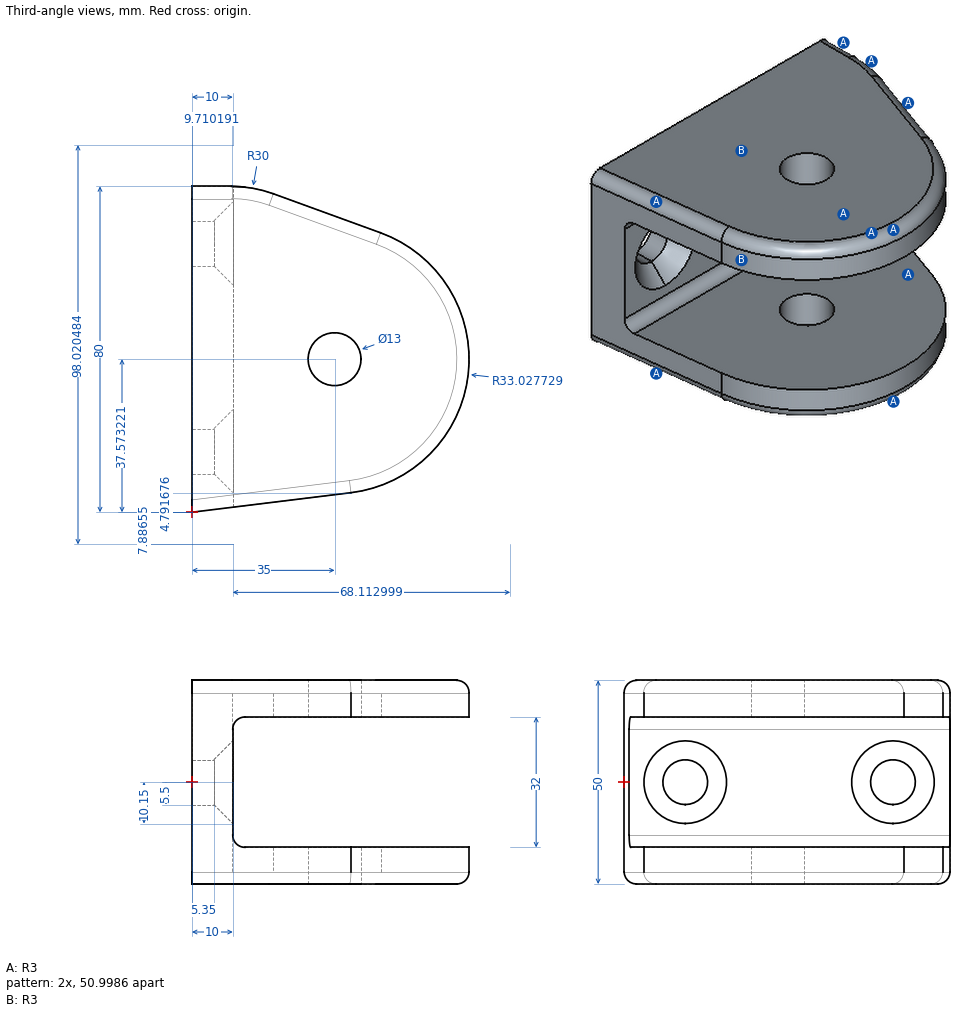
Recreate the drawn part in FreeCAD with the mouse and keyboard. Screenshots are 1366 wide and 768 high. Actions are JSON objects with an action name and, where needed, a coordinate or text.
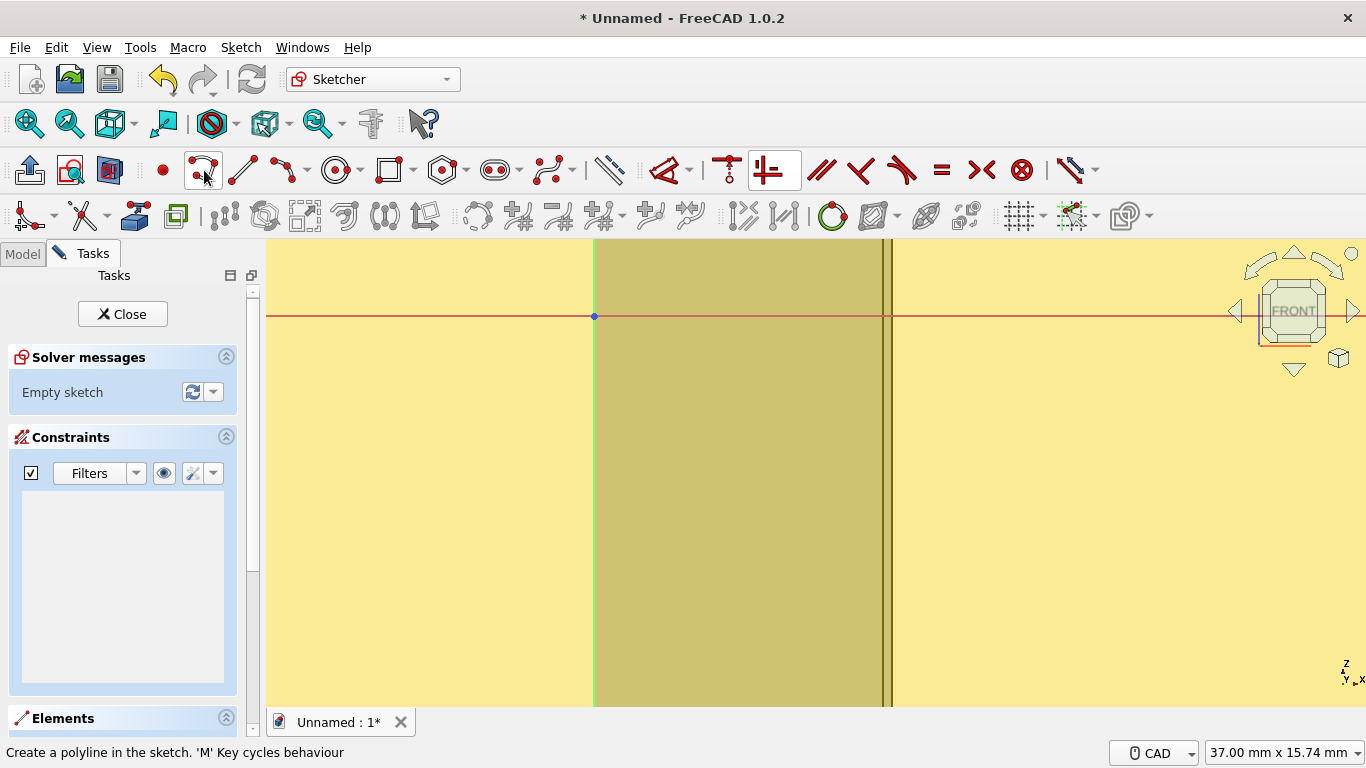
{"action": "left_click", "coordinate": [594, 316]}
{"action": "left_click", "coordinate": [892, 325]}
{"action": "left_click", "coordinate": [892, 618]}
{"action": "left_click", "coordinate": [754, 480]}
{"action": "left_click", "coordinate": [603, 480]}
{"action": "left_click", "coordinate": [594, 316]}
{"action": "key", "text": "Escape"}
{"action": "key", "text": "Escape"}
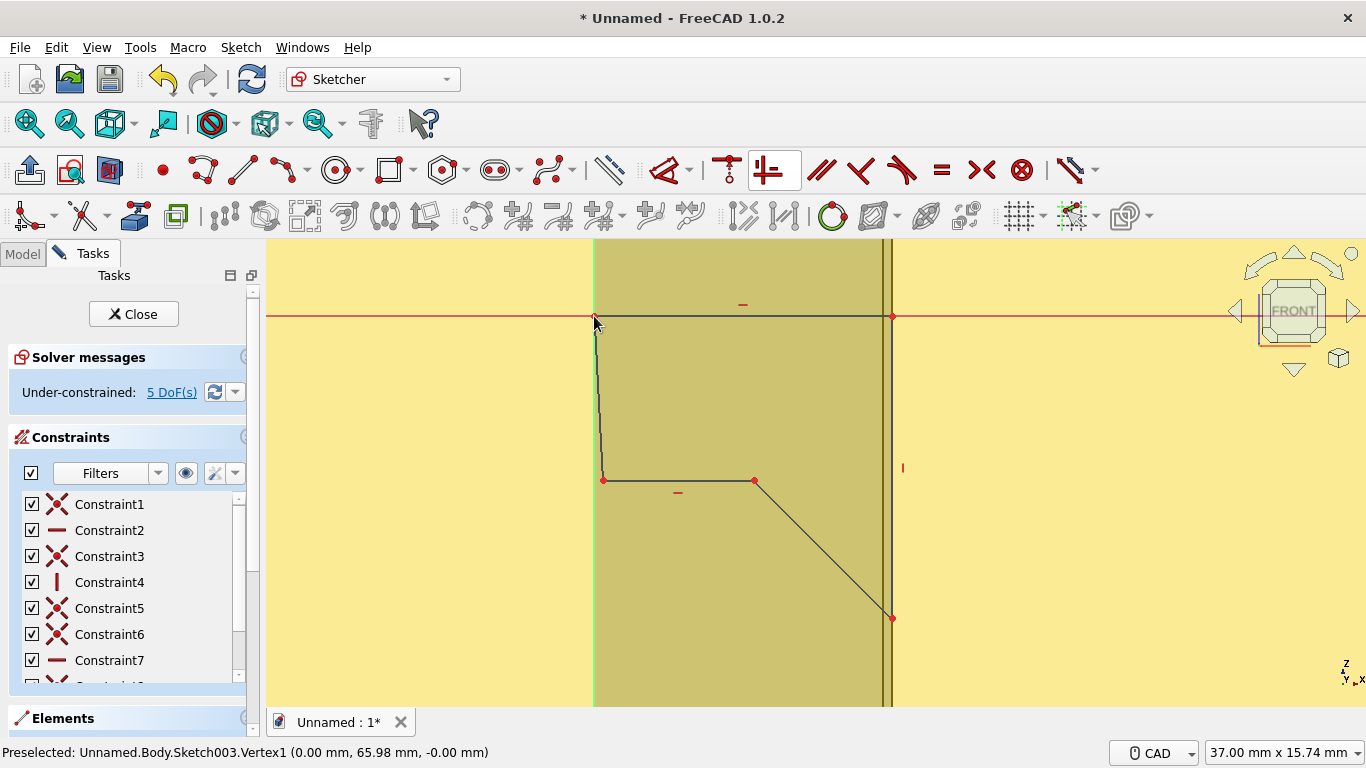
{"action": "left_click", "coordinate": [597, 366]}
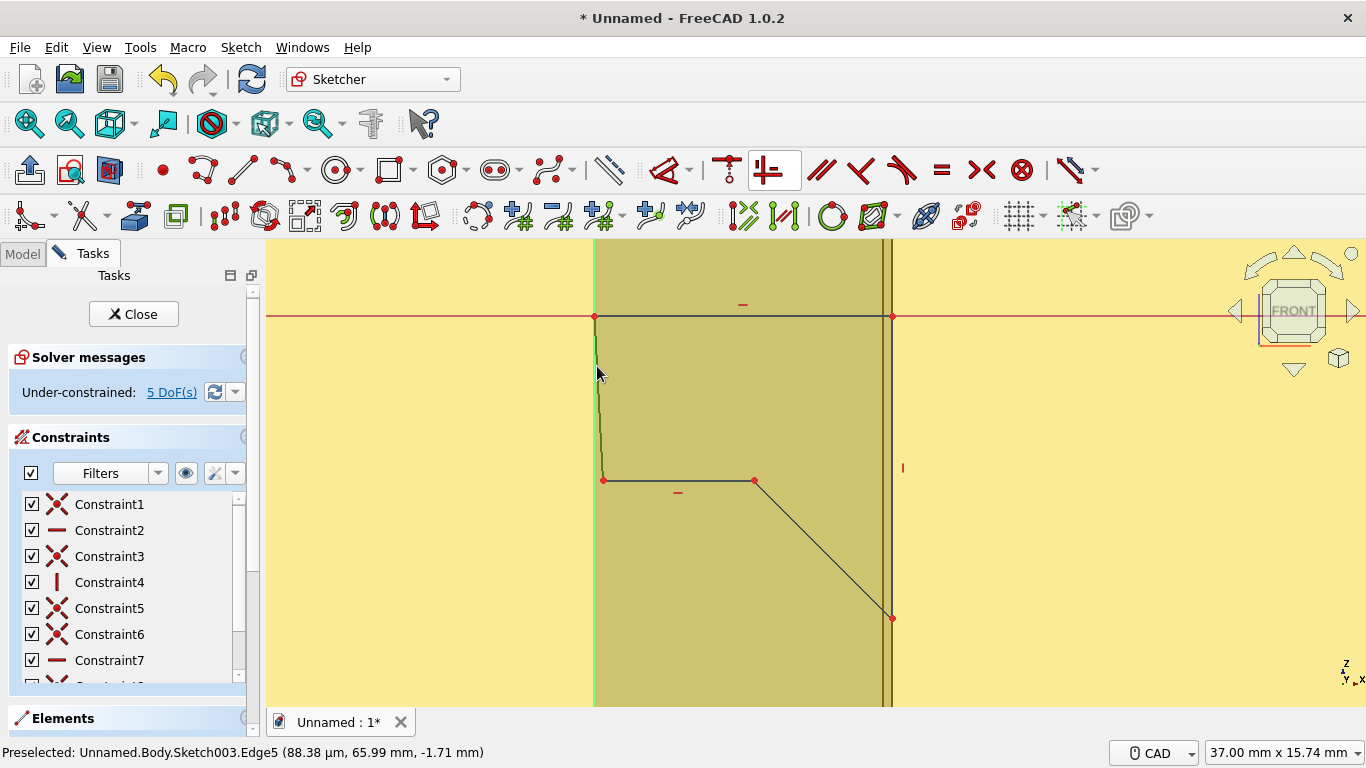
{"action": "left_click", "coordinate": [796, 170]}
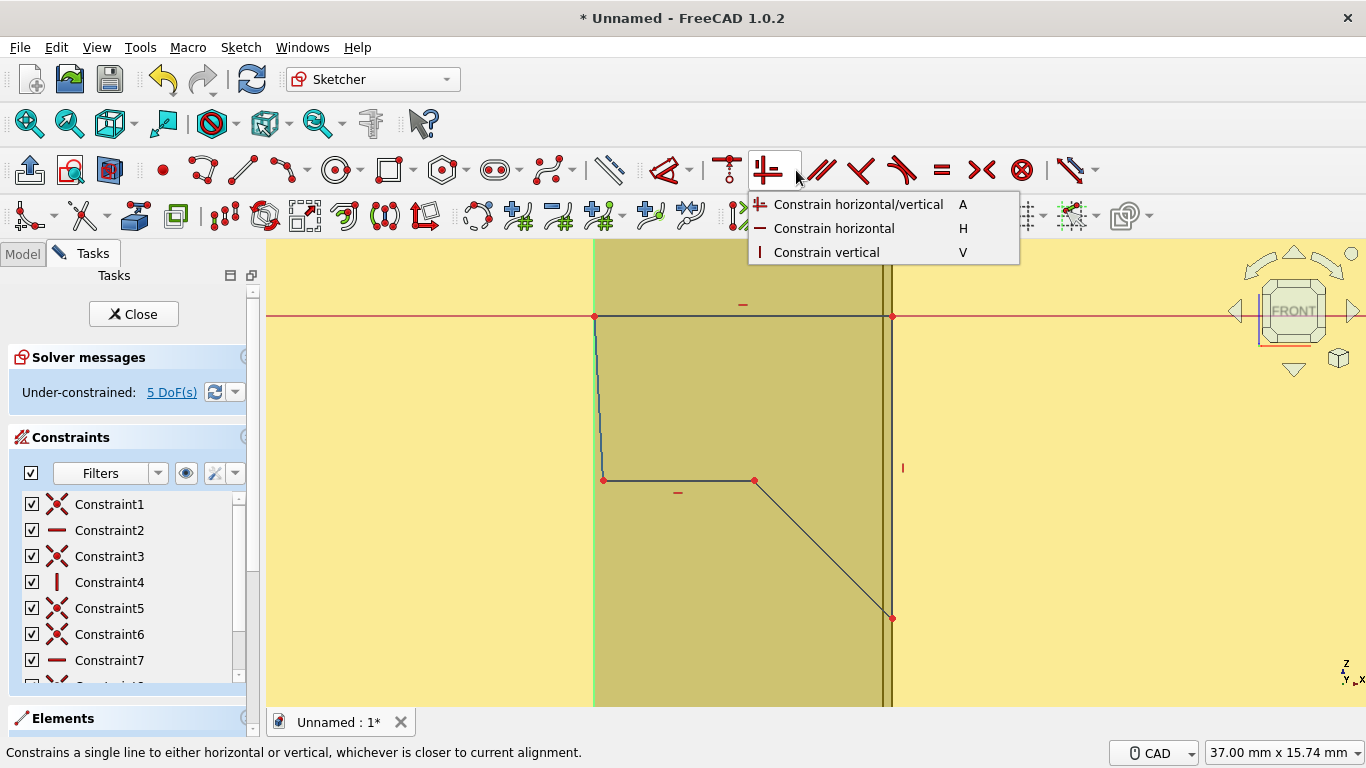
{"action": "left_click", "coordinate": [884, 252]}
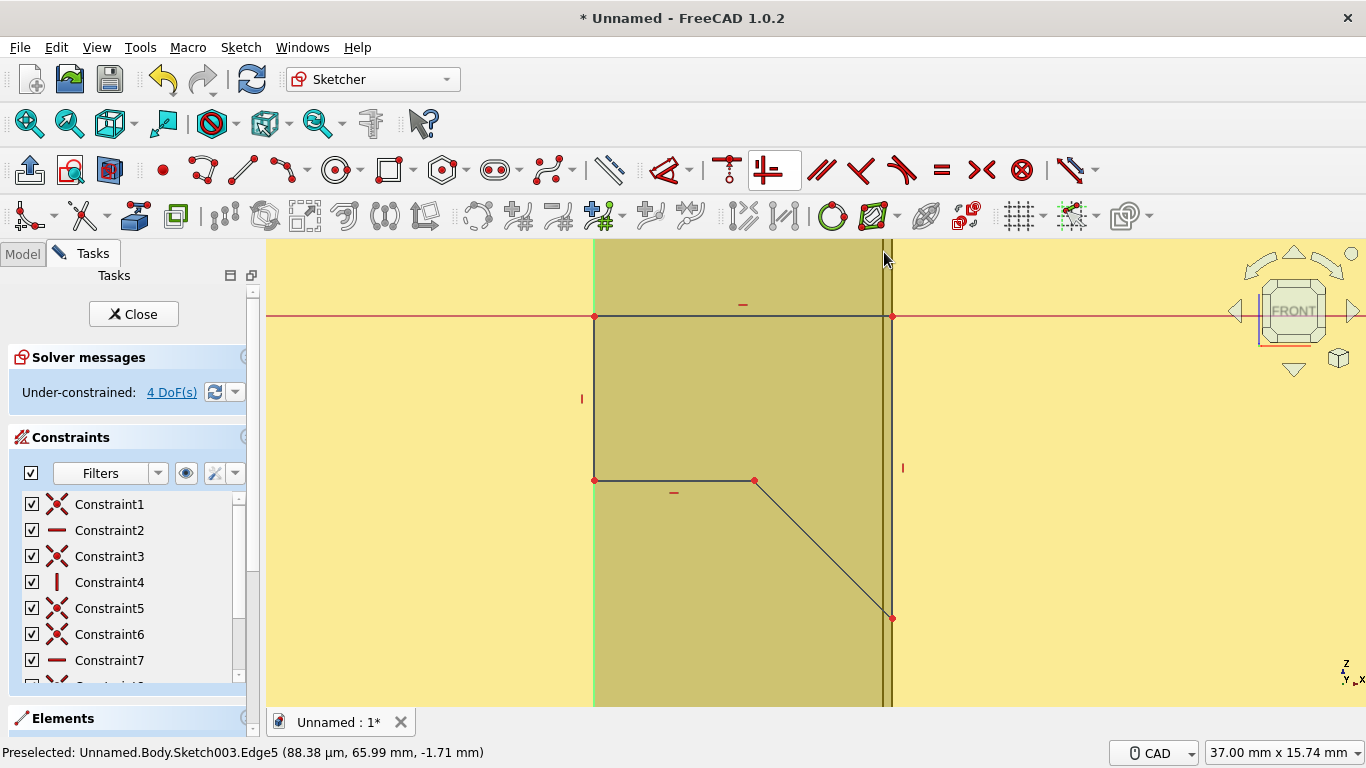
{"action": "left_click", "coordinate": [664, 170]}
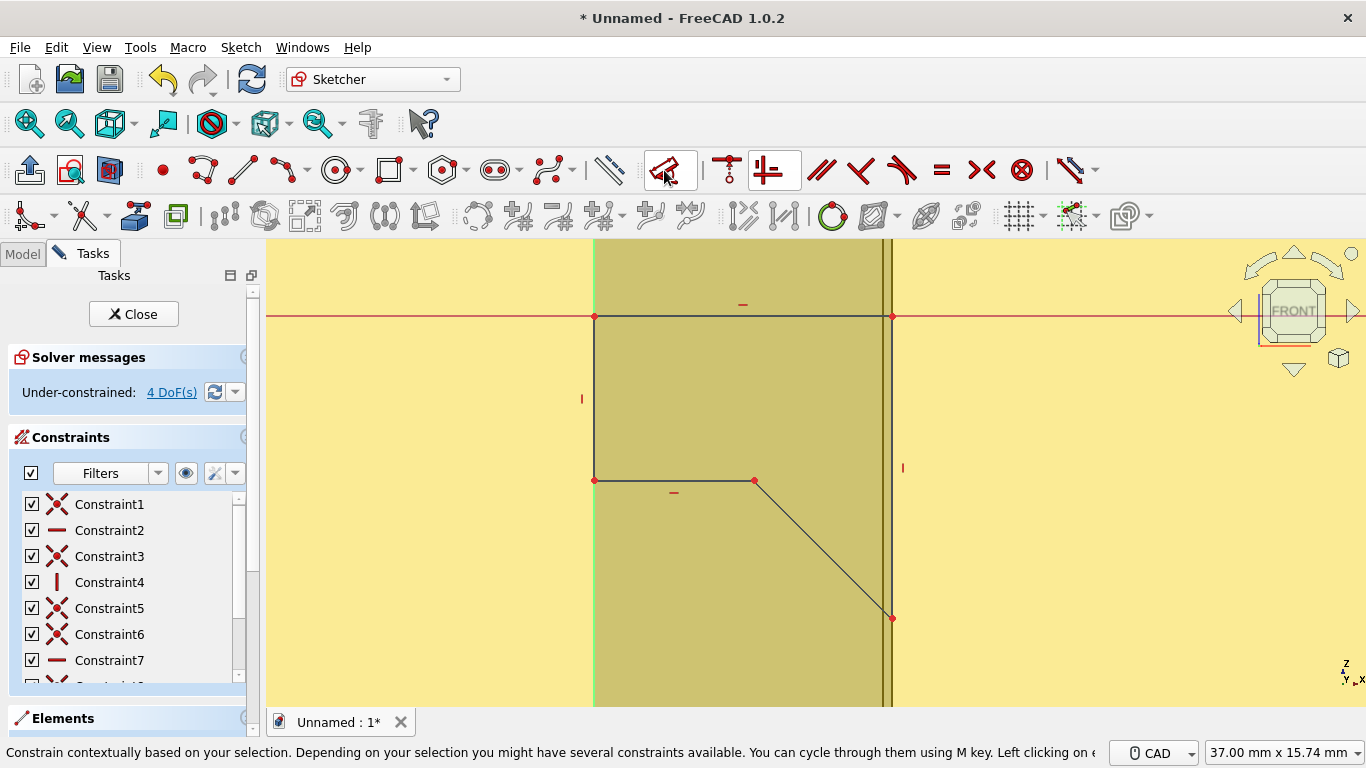
{"action": "left_click", "coordinate": [684, 316]}
{"action": "left_click", "coordinate": [743, 282]}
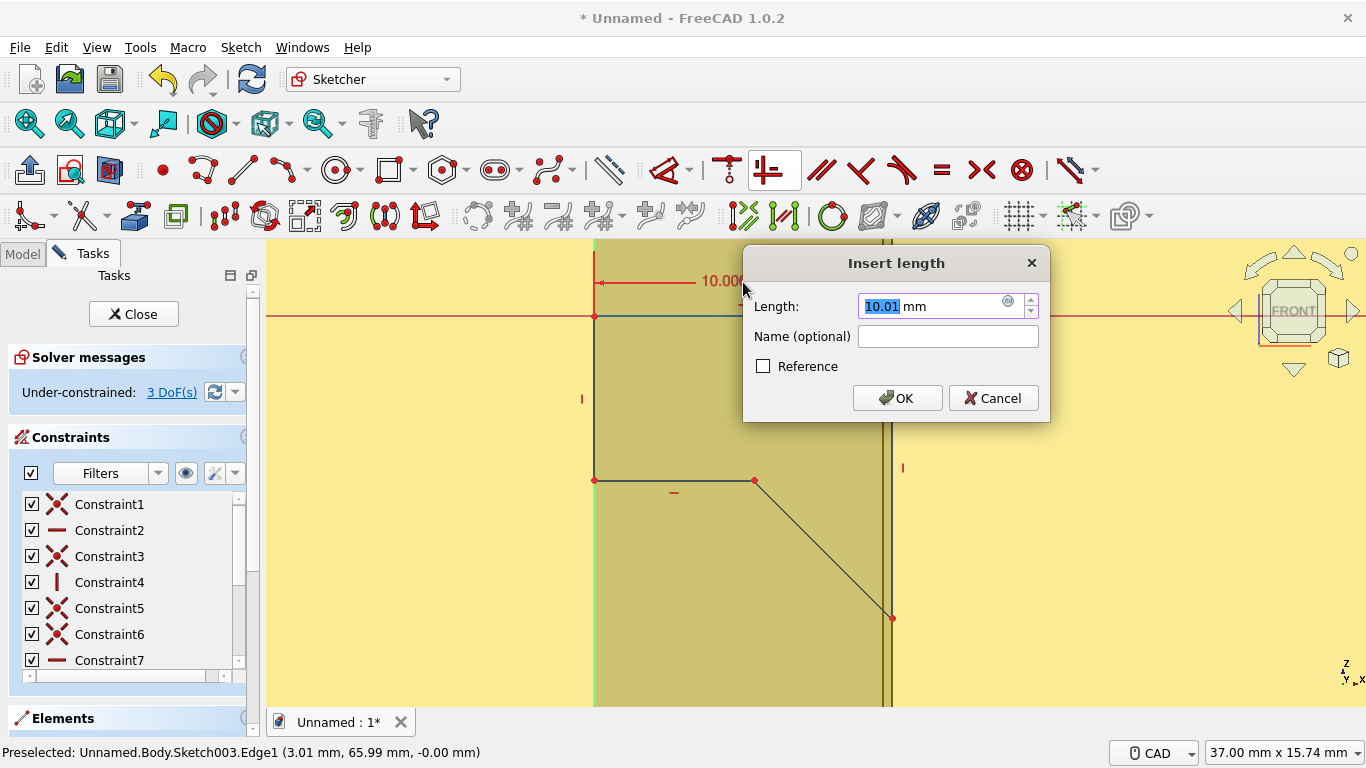
{"action": "type", "text": "10"}
{"action": "key", "text": "Return"}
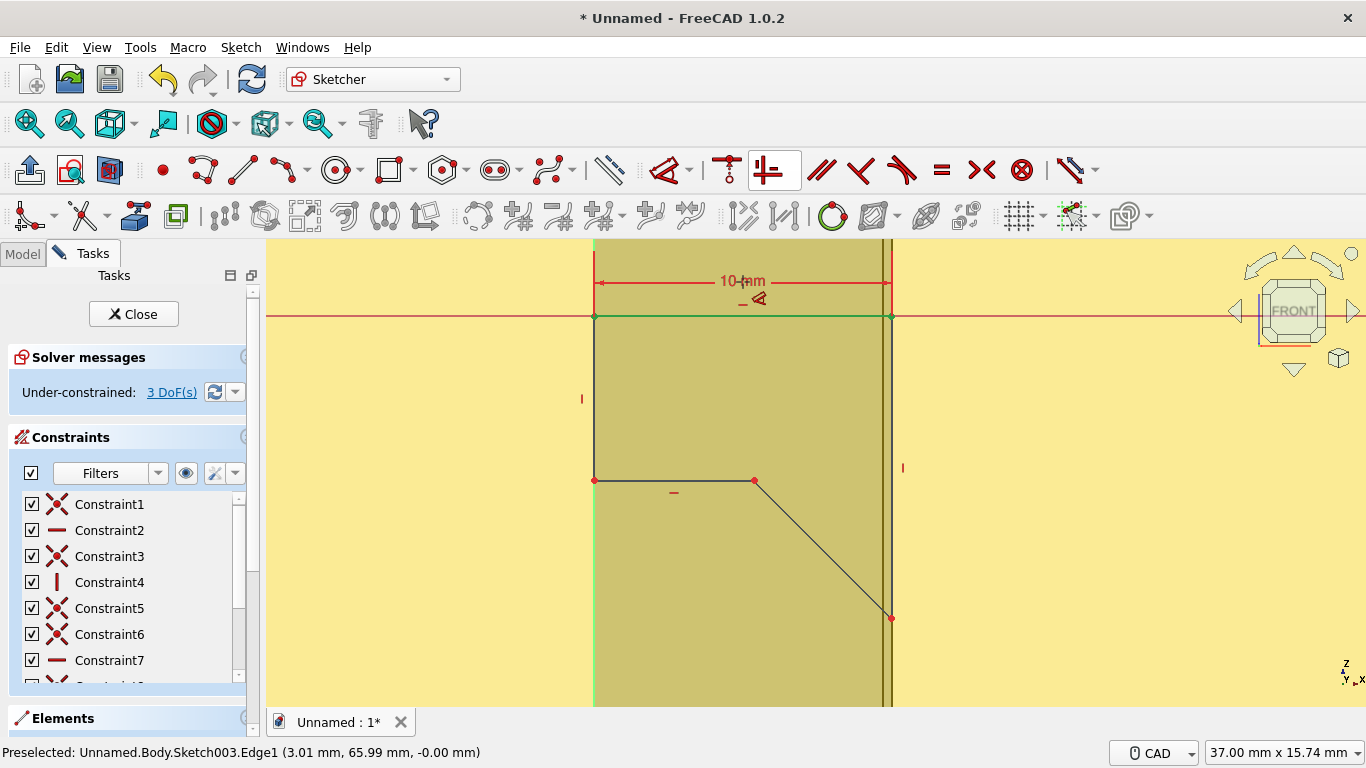
{"action": "left_click", "coordinate": [594, 432]}
{"action": "left_click", "coordinate": [560, 399]}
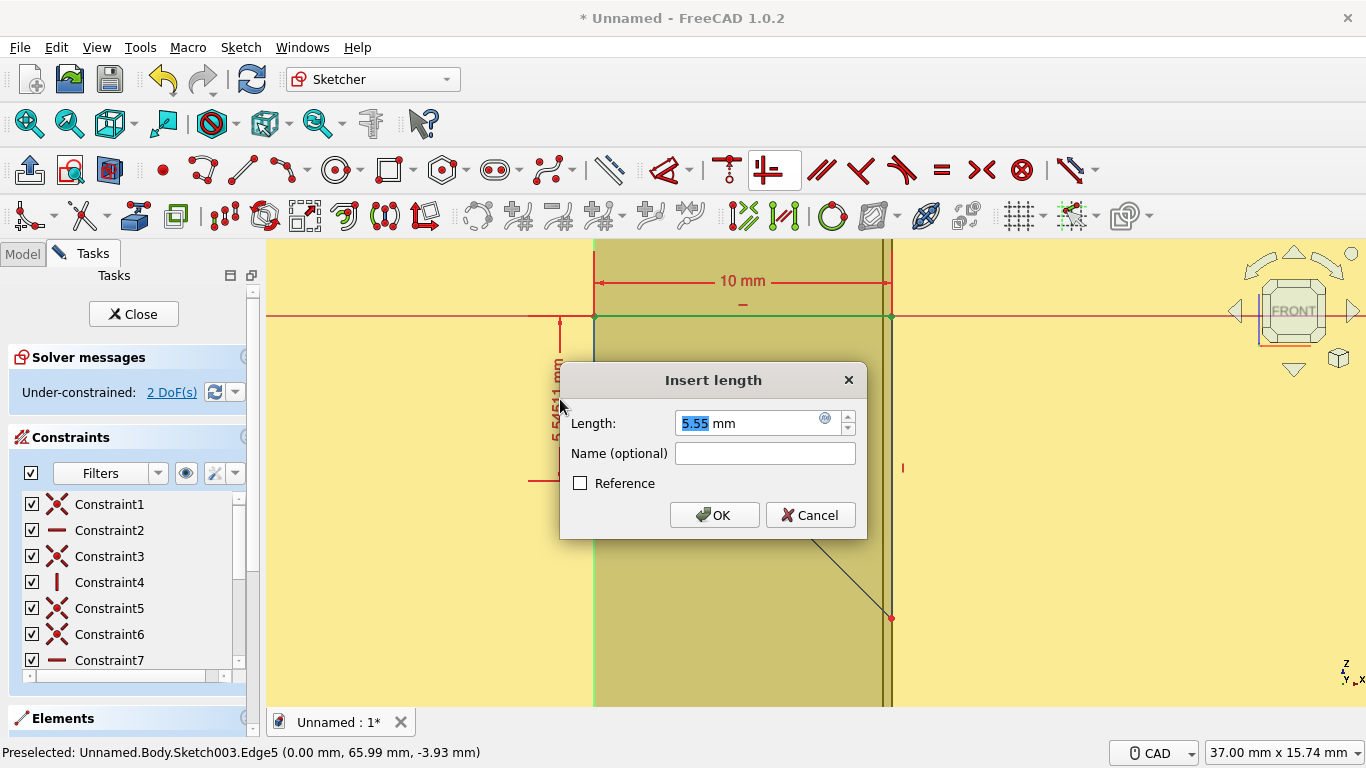
{"action": "type", "text": "5.5"}
{"action": "key", "text": "Return"}